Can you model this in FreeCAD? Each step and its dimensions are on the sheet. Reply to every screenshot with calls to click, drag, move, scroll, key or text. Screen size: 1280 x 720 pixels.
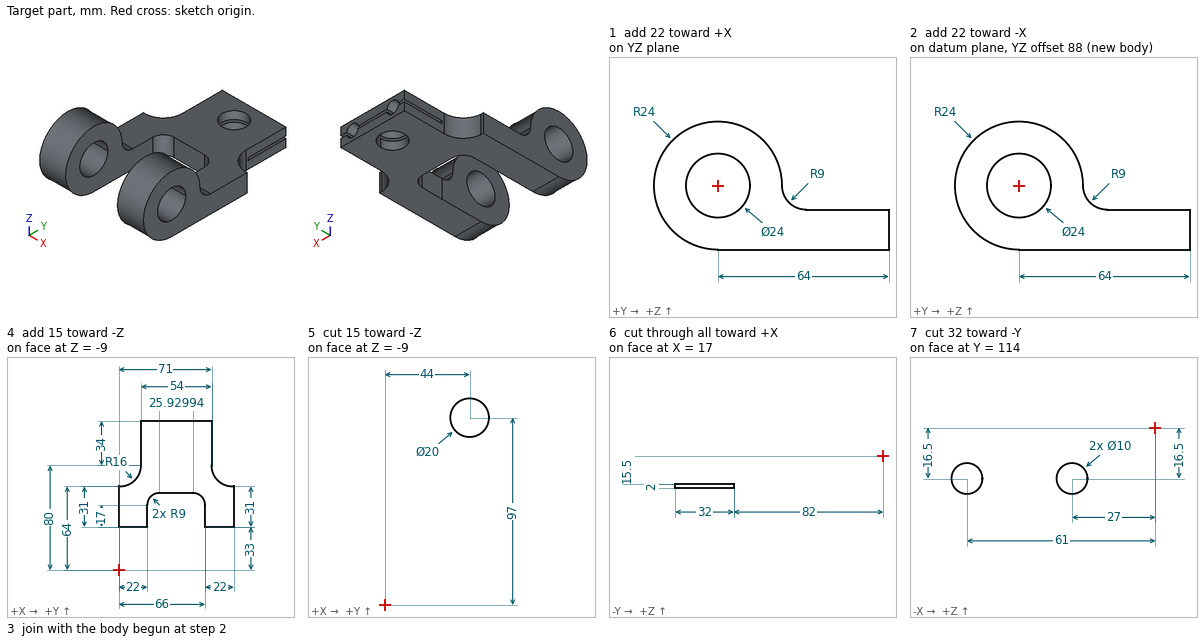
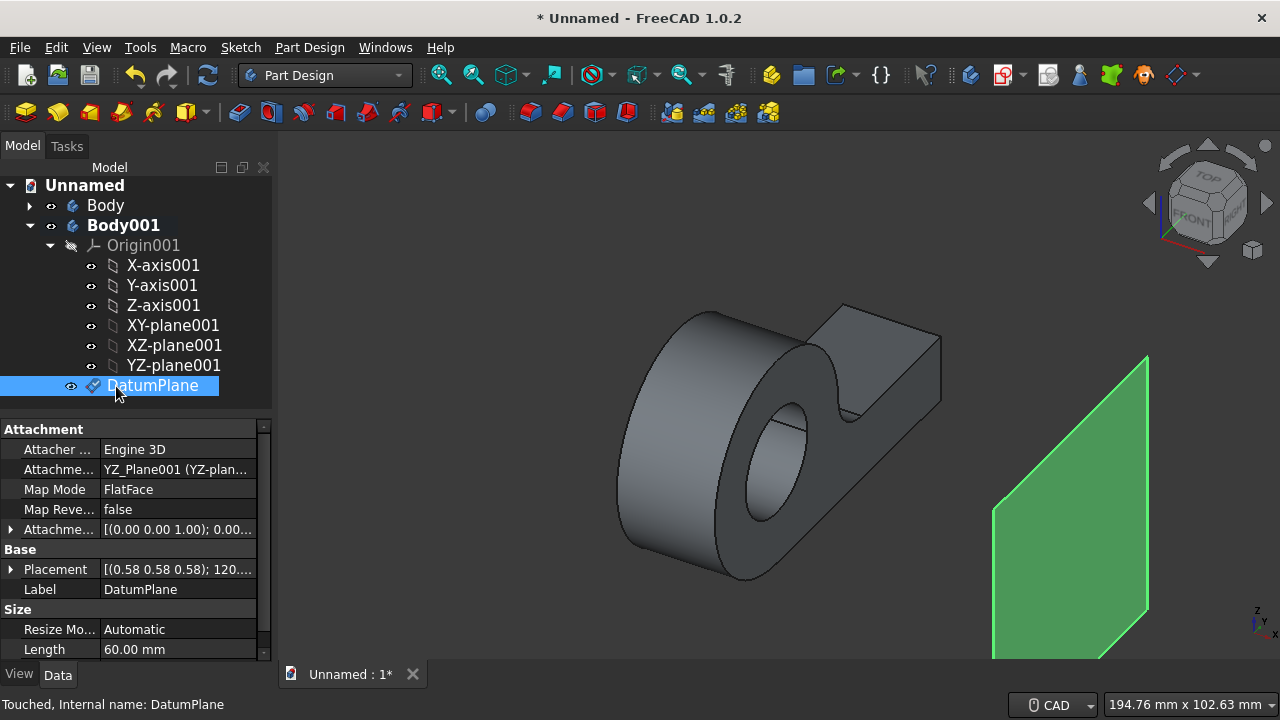
click(1004, 76)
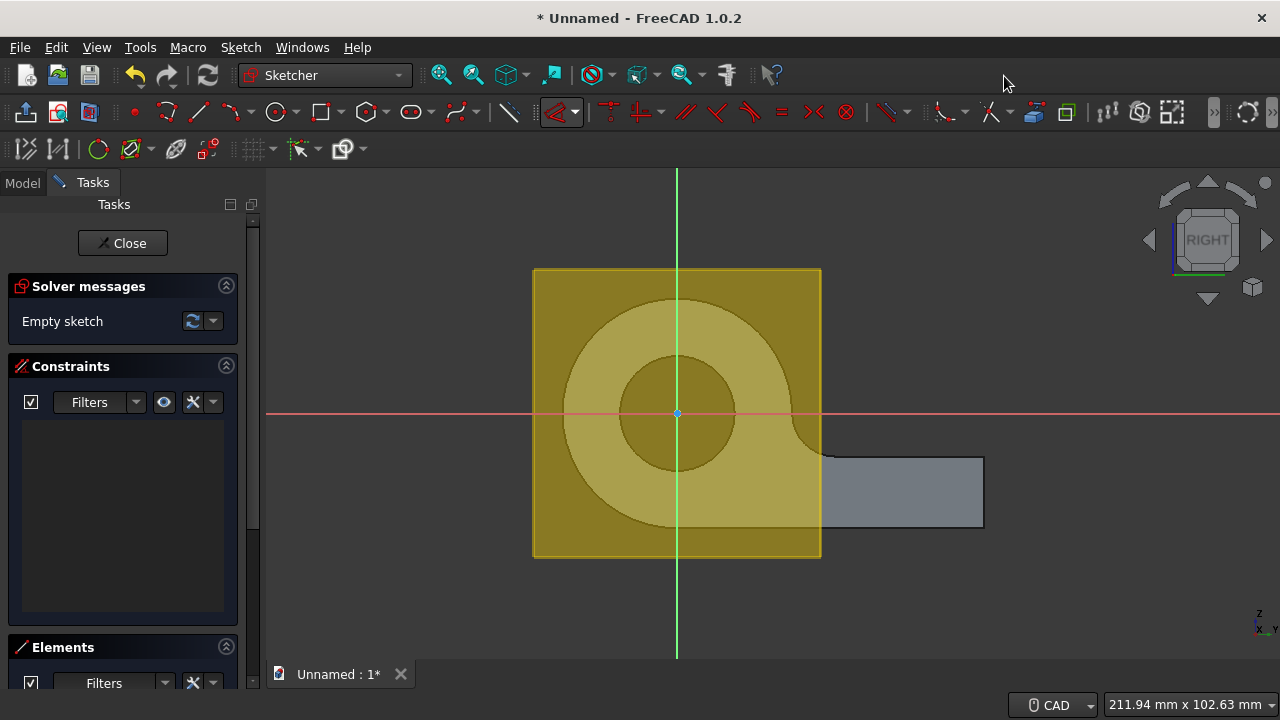
scroll(963, 465, up, 2)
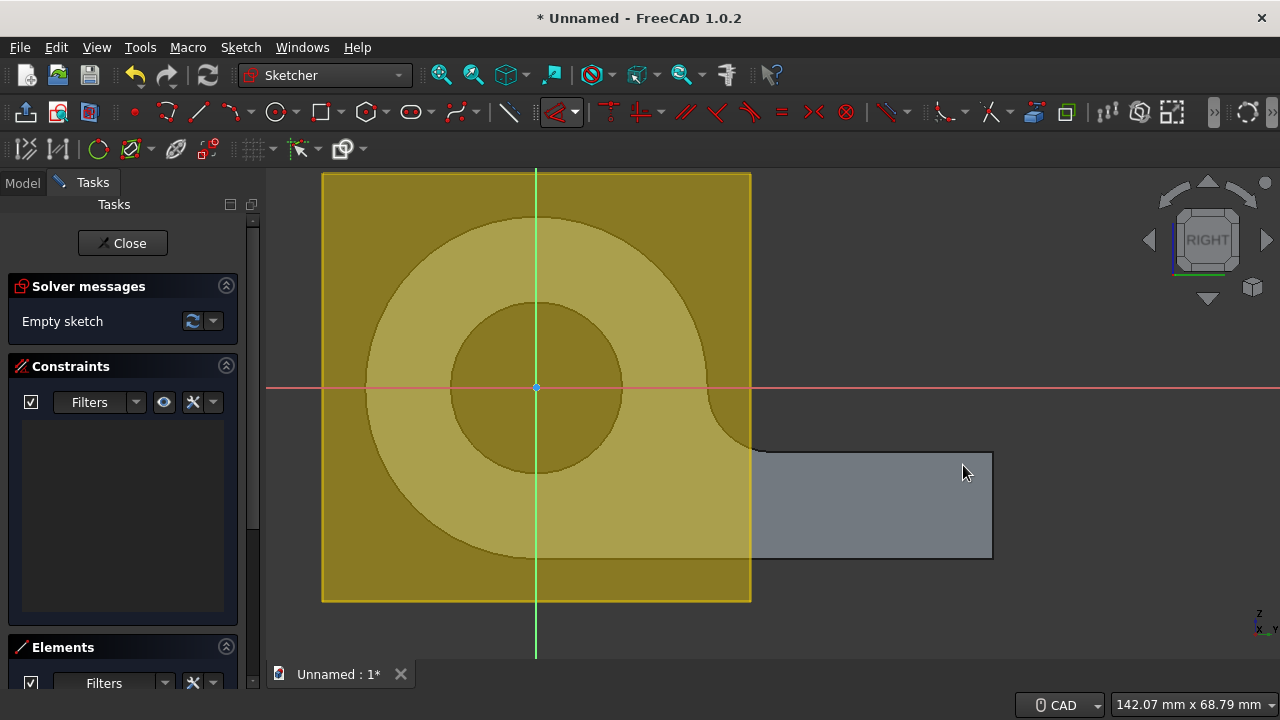
click(168, 112)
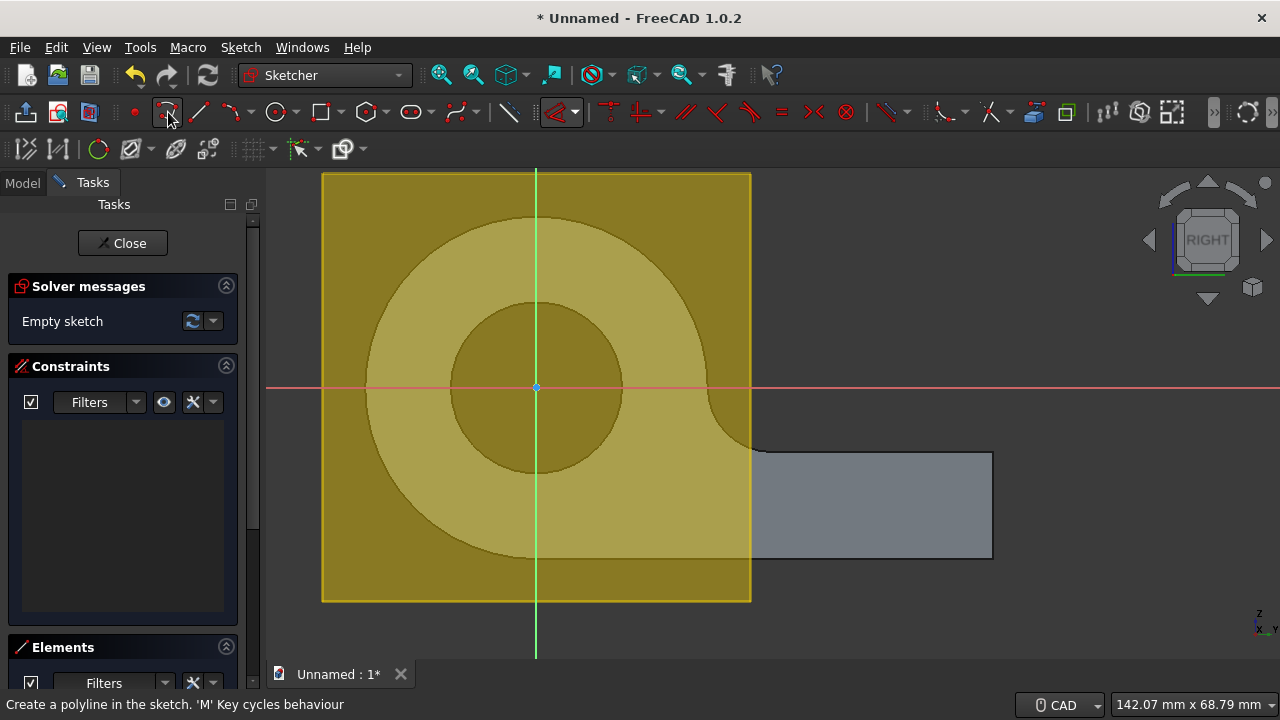
click(536, 559)
click(993, 559)
click(993, 452)
click(772, 452)
right_click(772, 452)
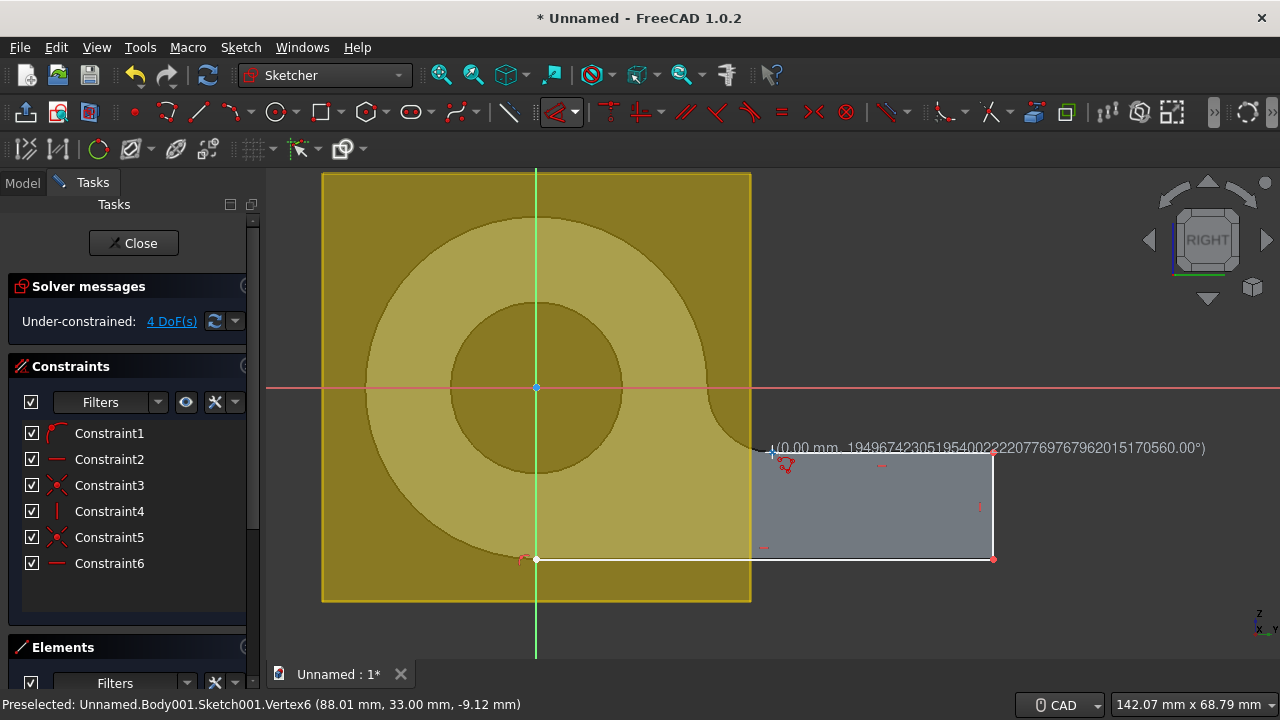
click(232, 112)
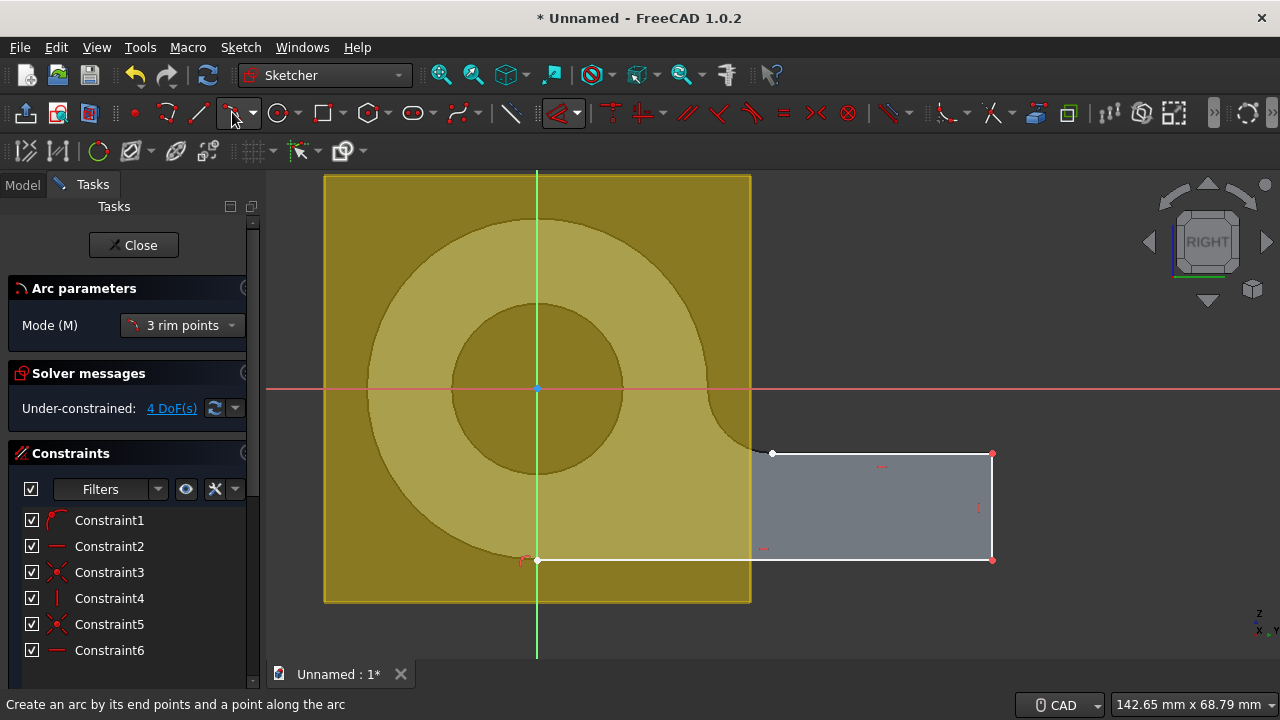
click(772, 454)
click(708, 389)
click(727, 434)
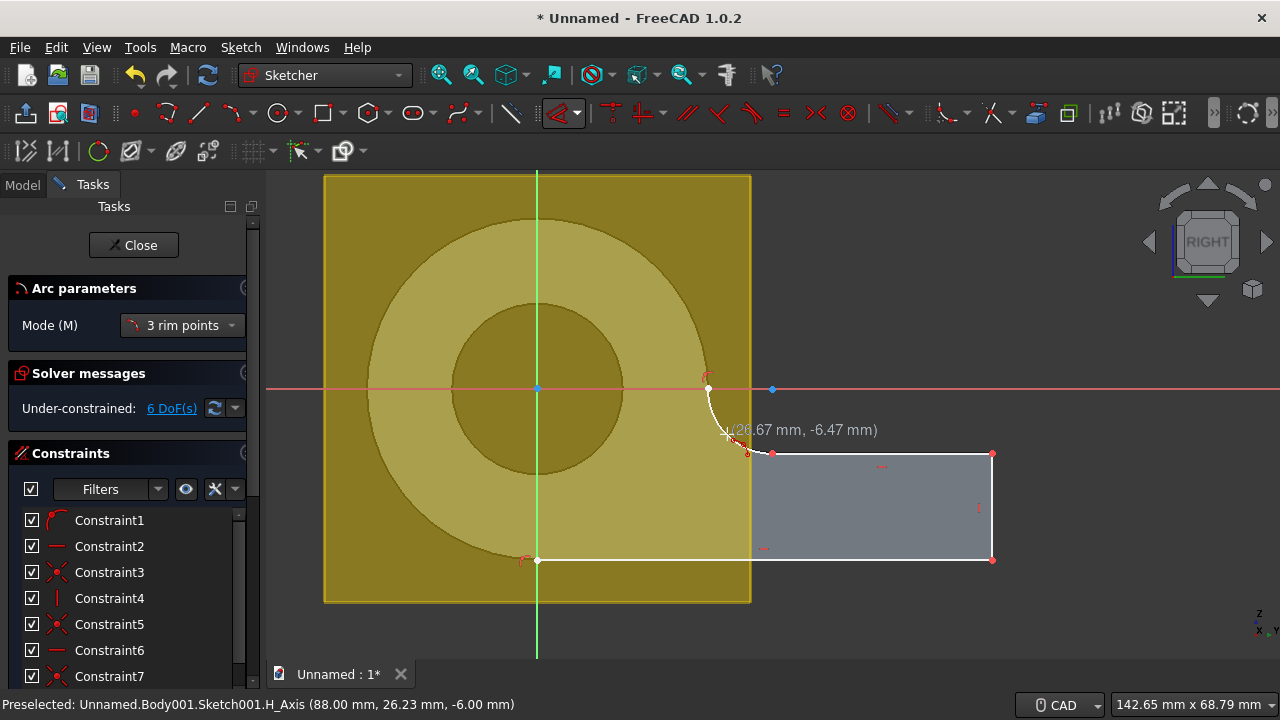
click(708, 389)
click(537, 560)
click(417, 268)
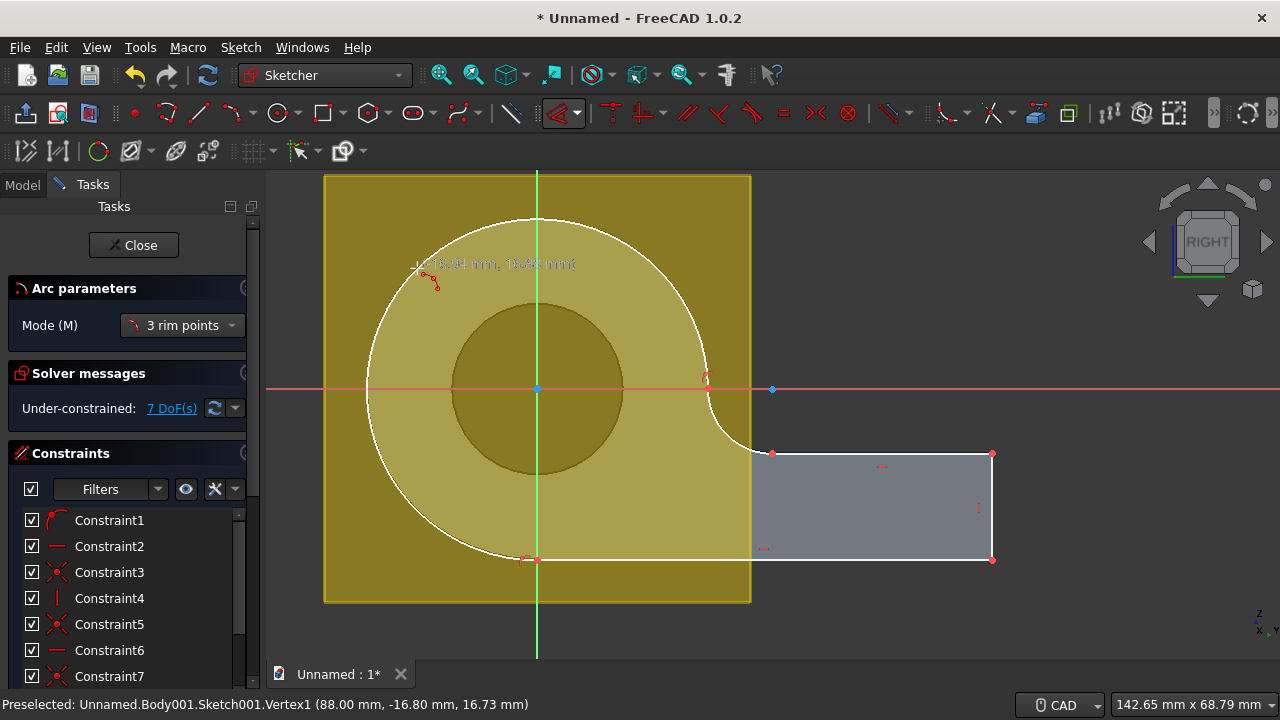
click(278, 114)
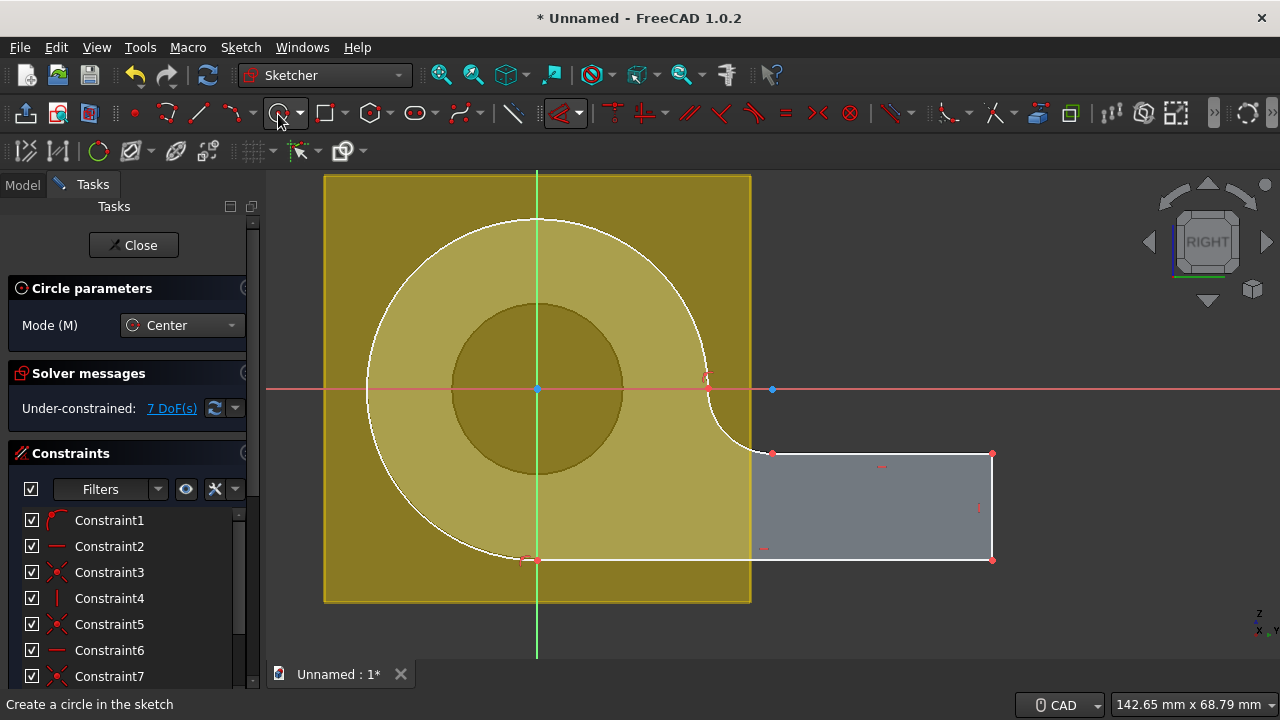
click(537, 389)
click(598, 329)
key(Escape)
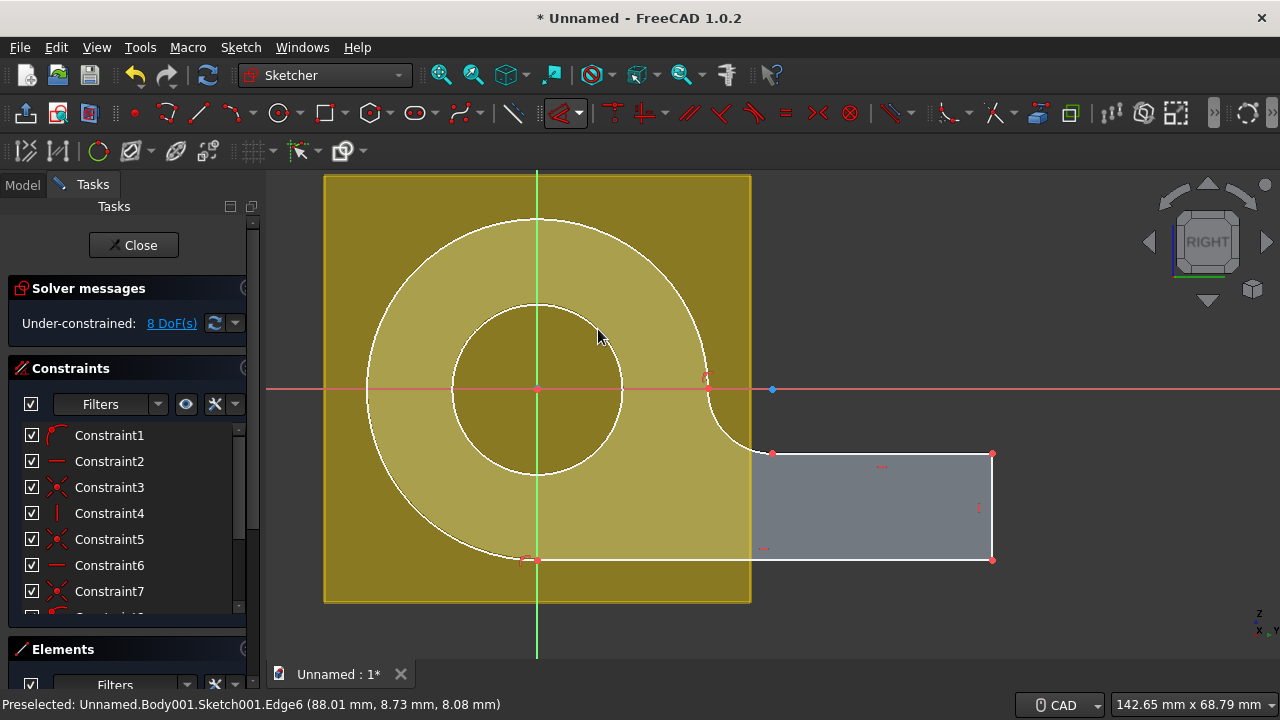
click(674, 560)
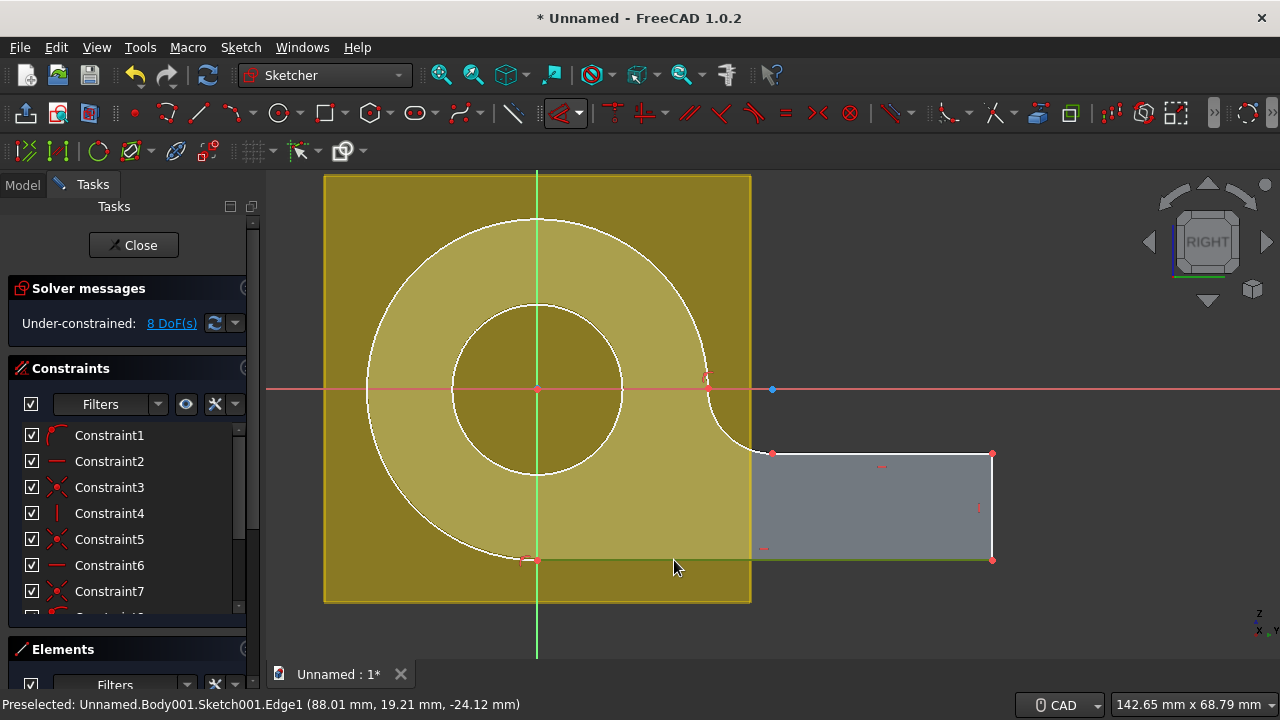
click(564, 221)